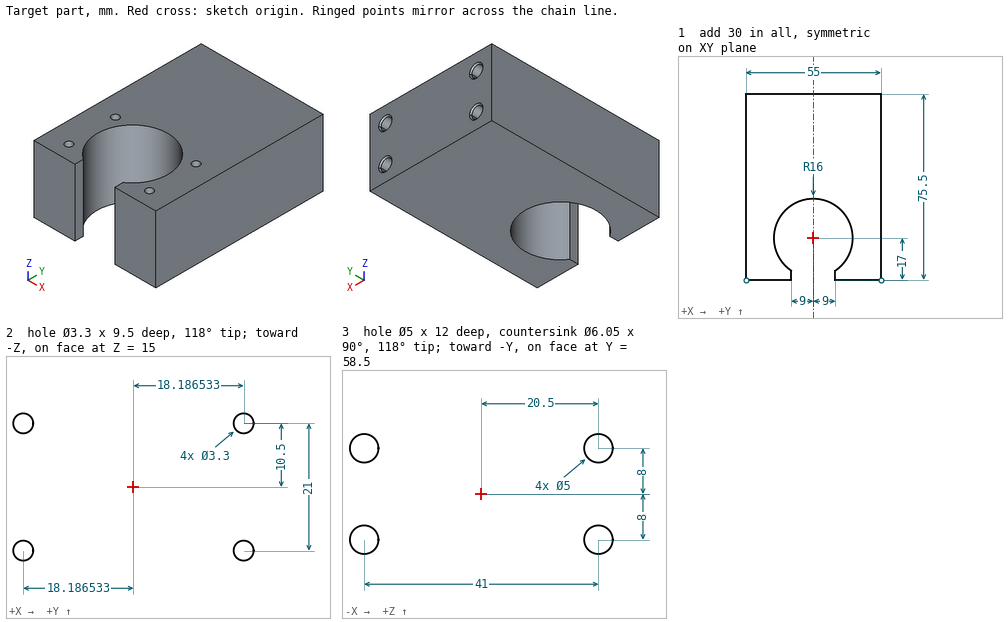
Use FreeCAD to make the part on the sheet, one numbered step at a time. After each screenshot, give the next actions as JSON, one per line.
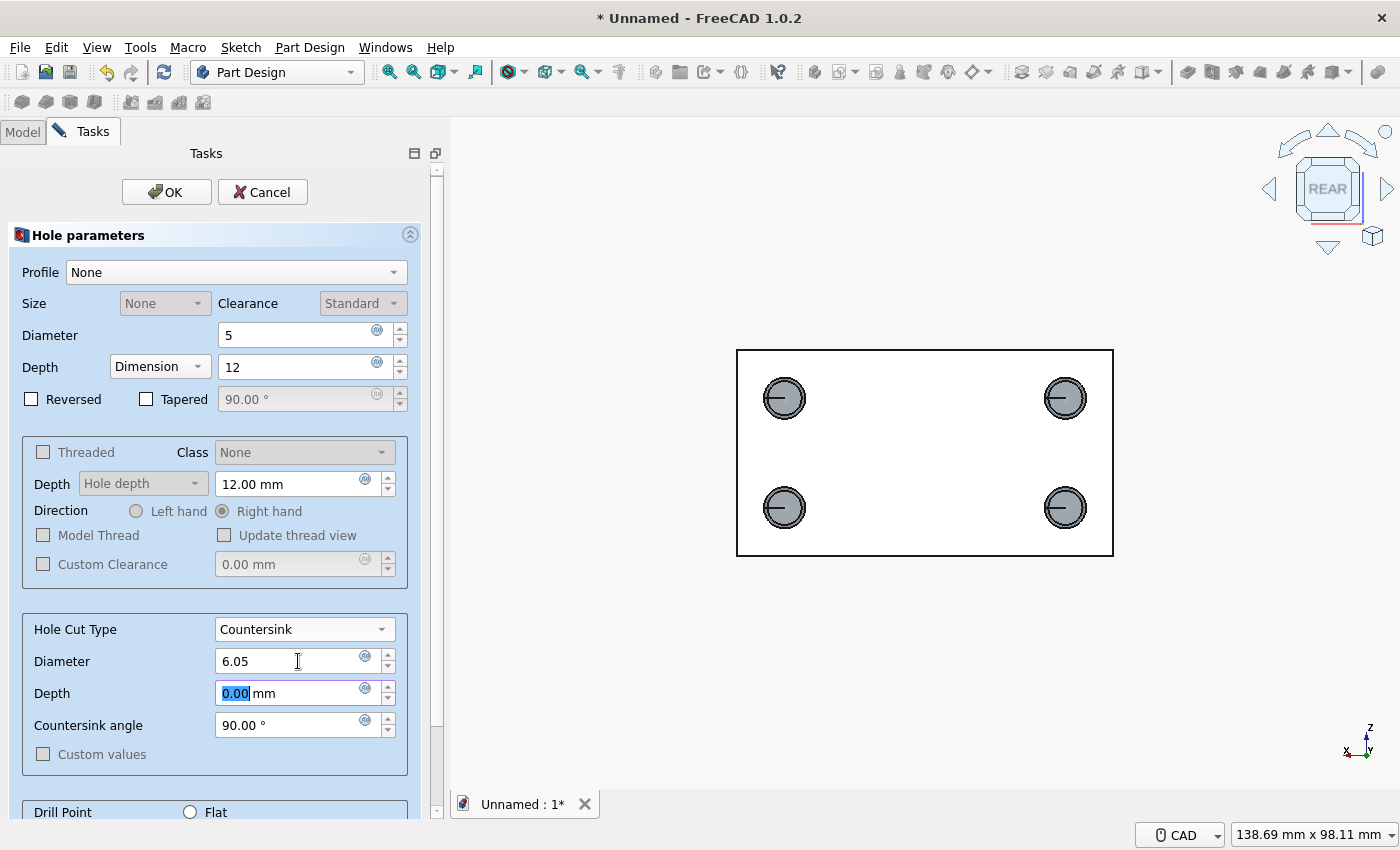
{"action": "left_click", "coordinate": [167, 192]}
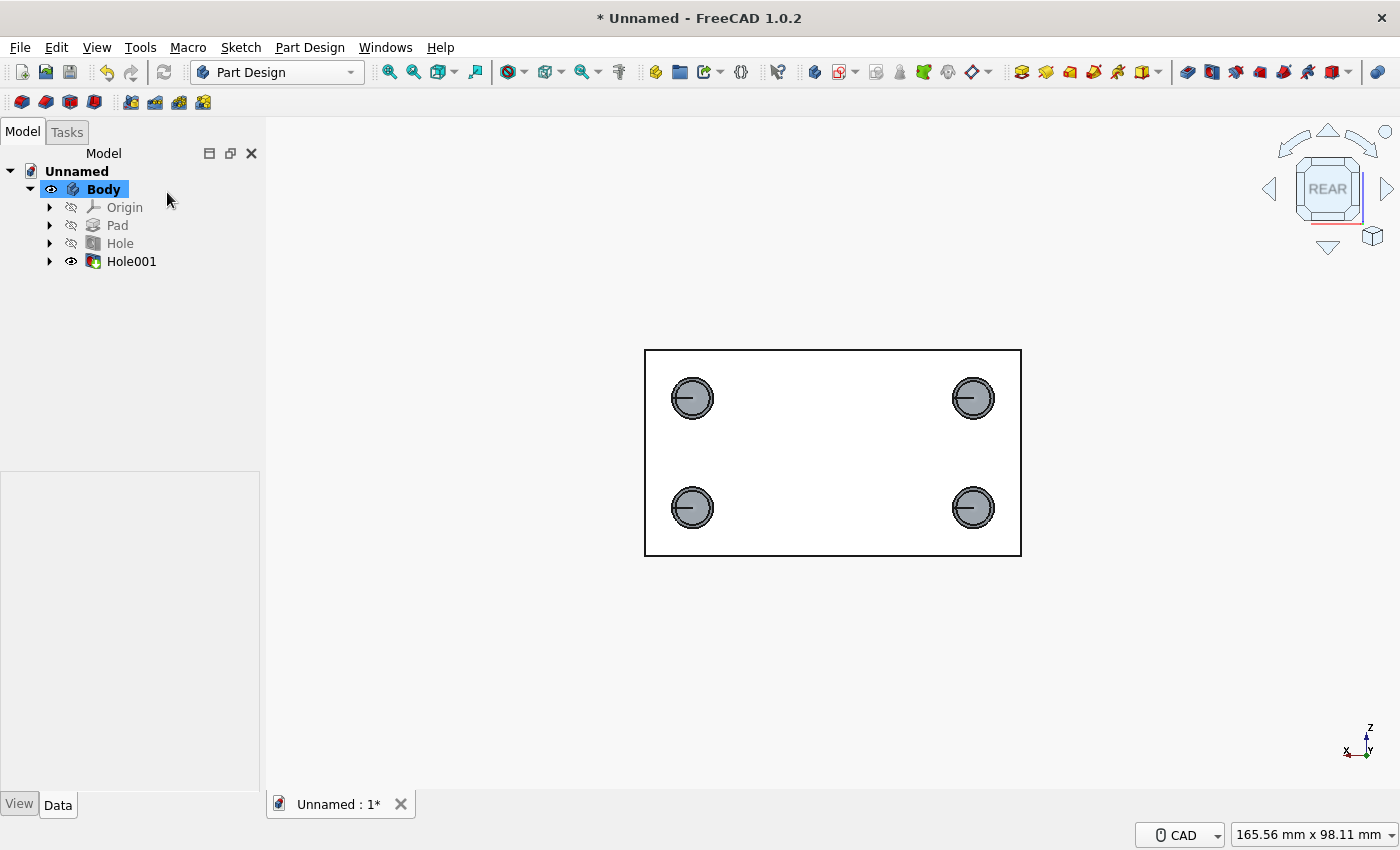
{"action": "key", "text": "0"}